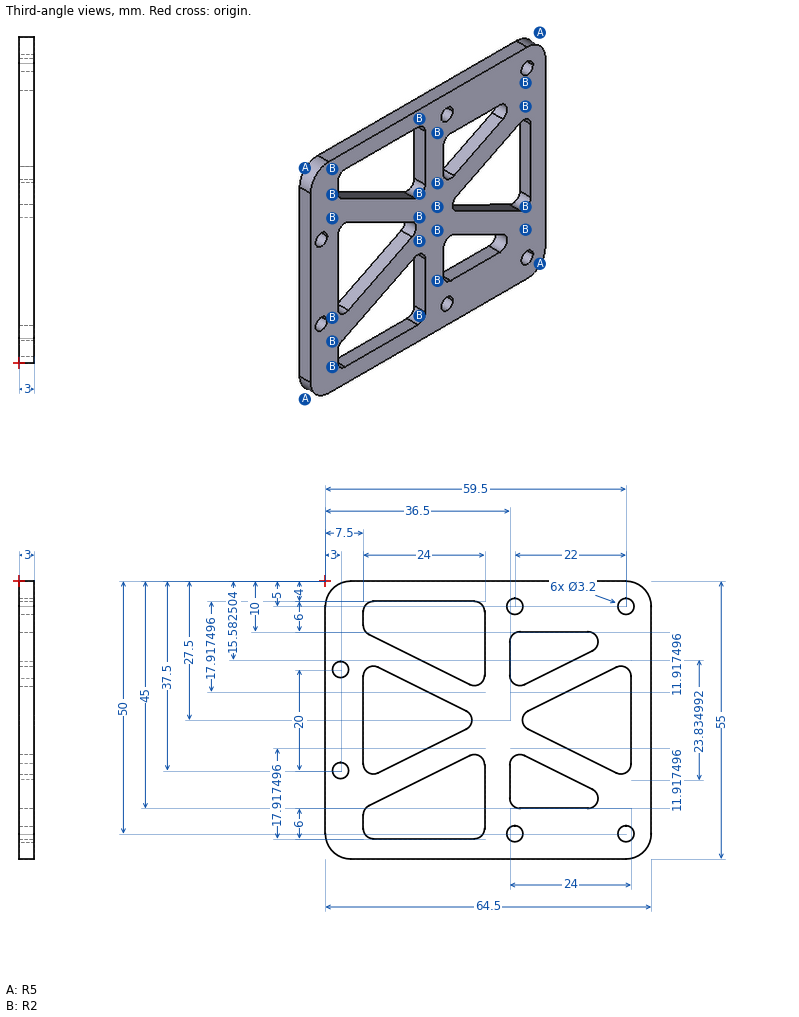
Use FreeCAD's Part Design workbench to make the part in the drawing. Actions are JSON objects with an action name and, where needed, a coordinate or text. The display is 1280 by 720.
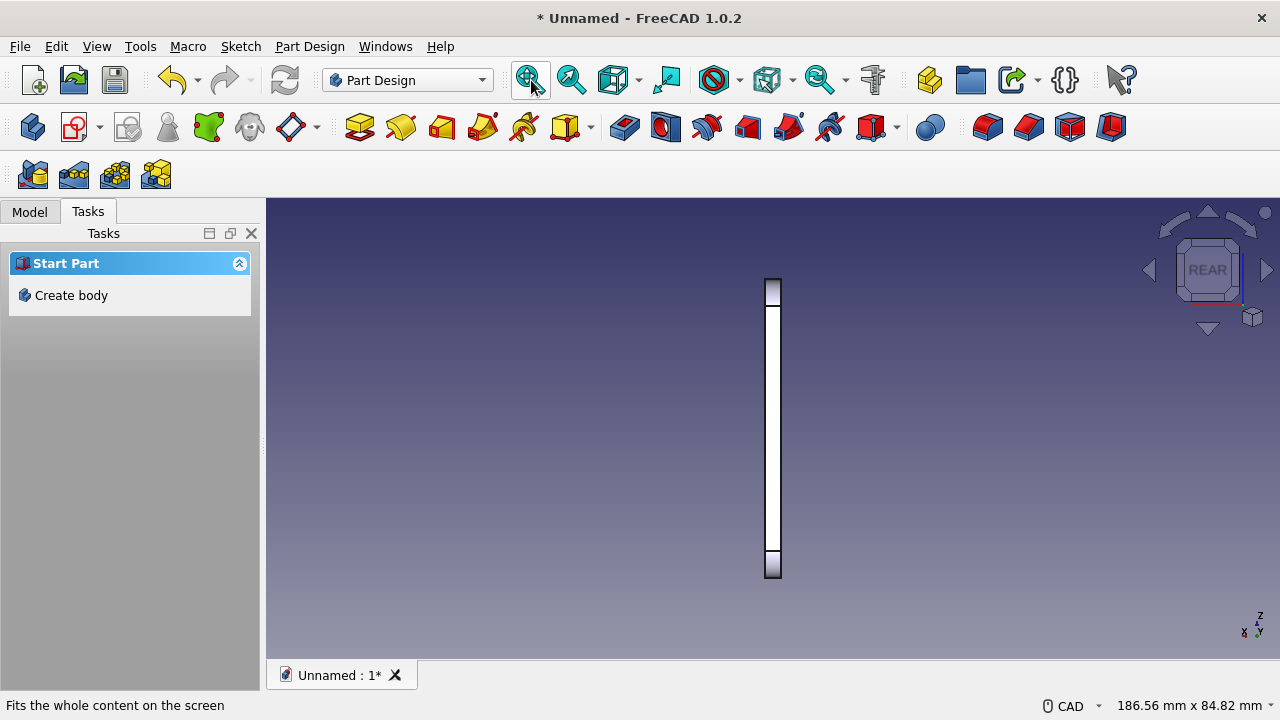
{"action": "scroll", "coordinate": [619, 523], "scroll_direction": "up", "scroll_amount": 5}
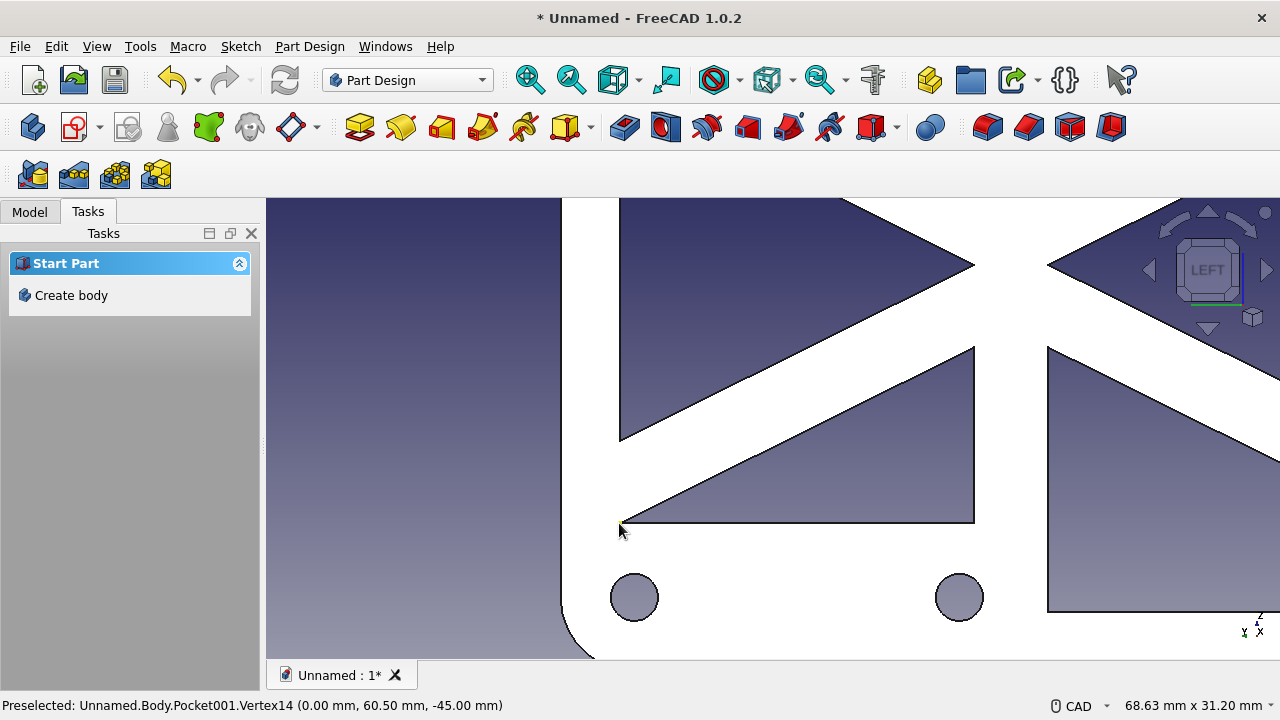
{"action": "key", "text": "v f"}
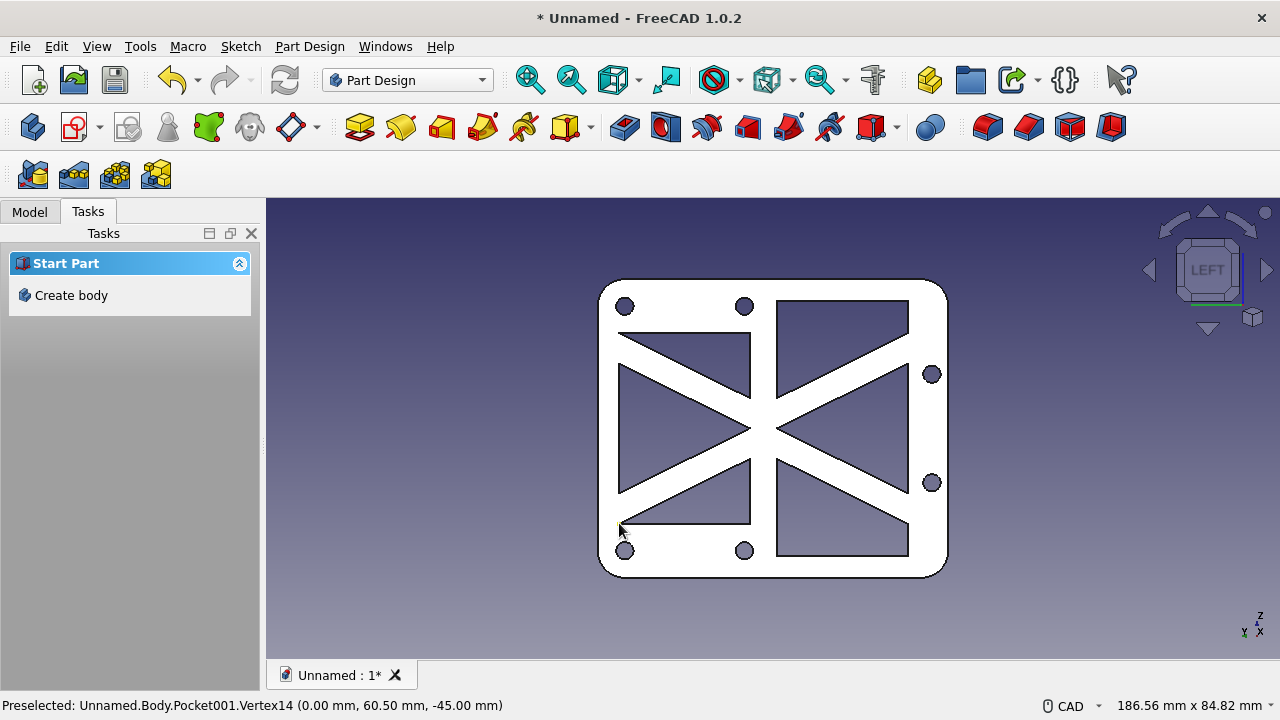
{"action": "key", "text": "v 3"}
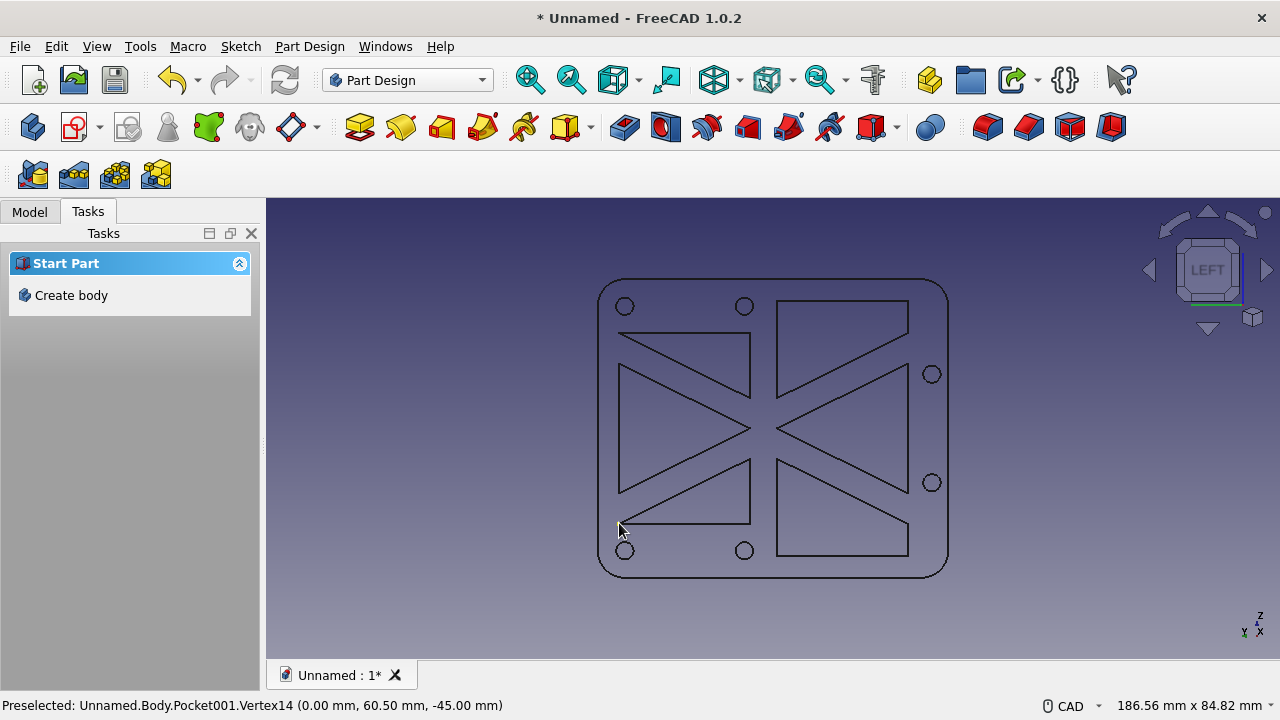
{"action": "key", "text": "0"}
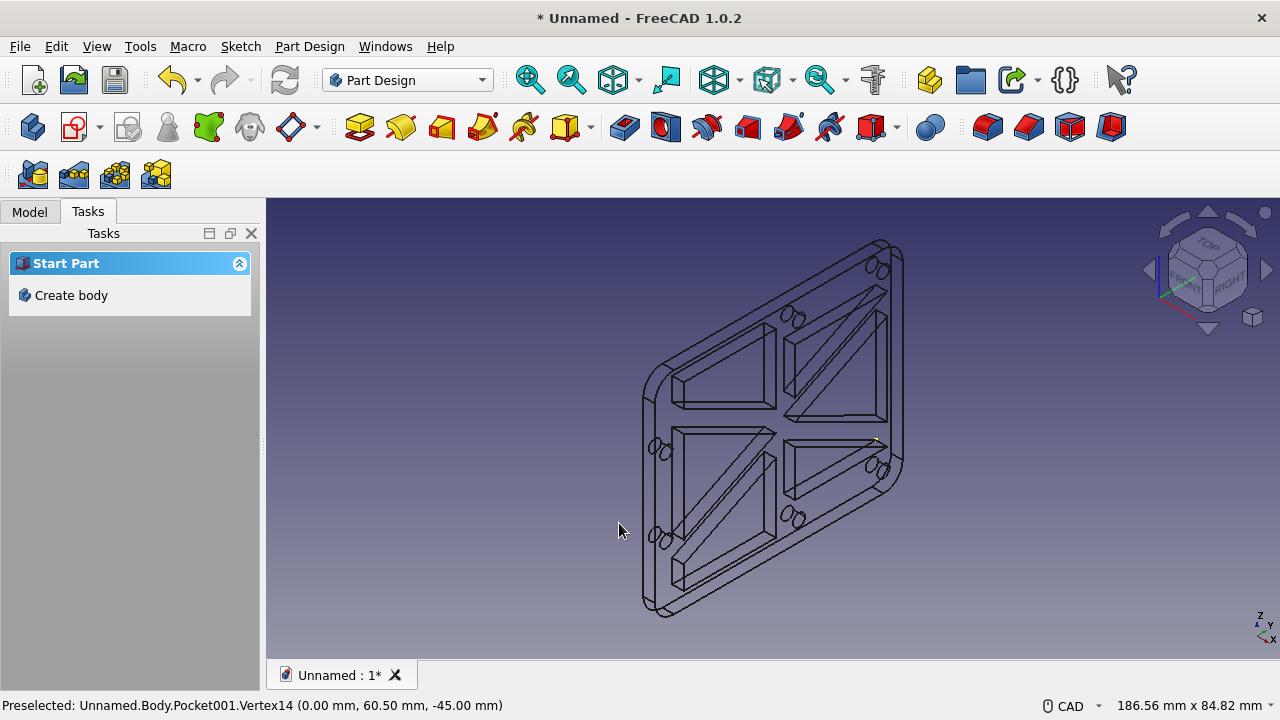
{"action": "left_click", "coordinate": [789, 443]}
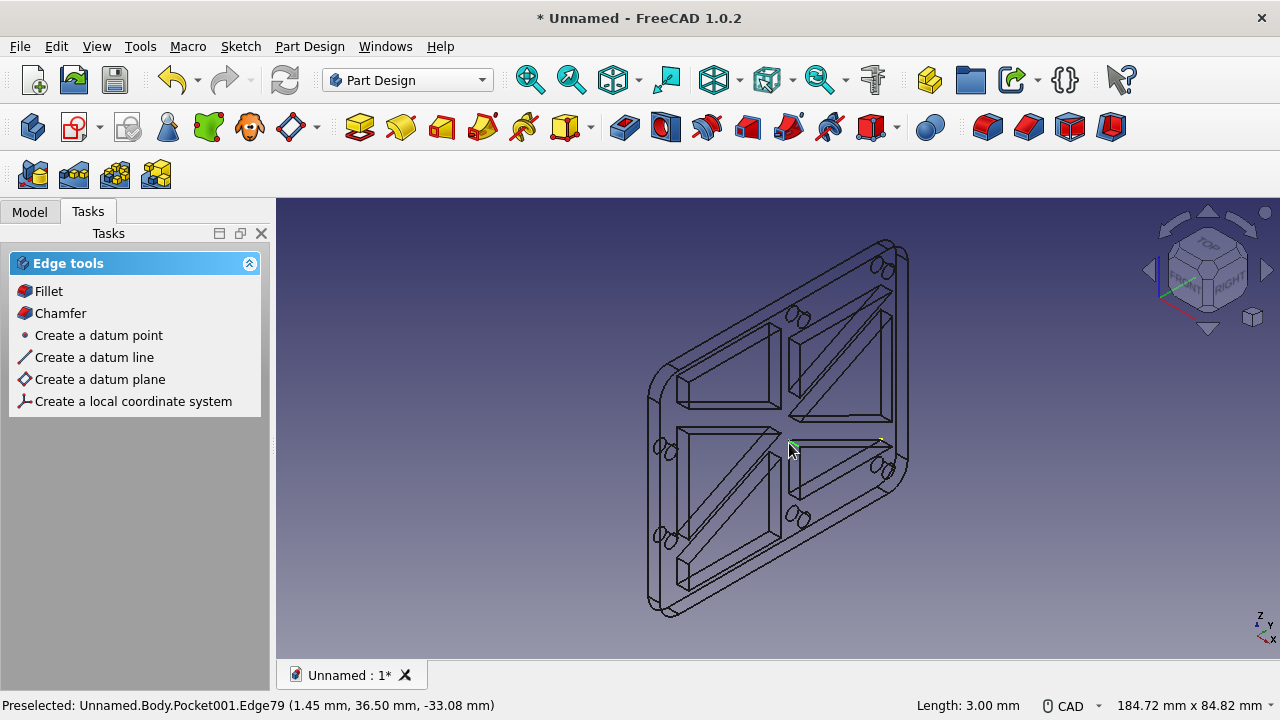
{"action": "left_click", "coordinate": [794, 496], "text": "ctrl"}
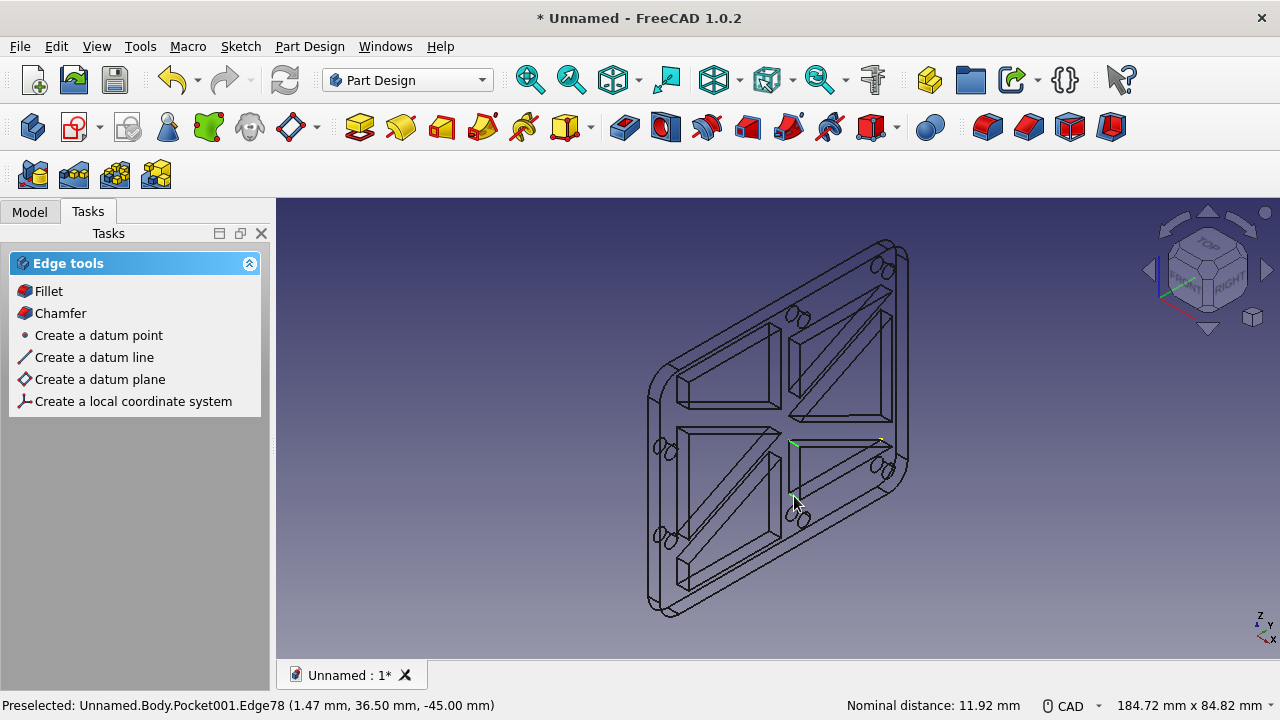
{"action": "left_click", "coordinate": [885, 311], "text": "ctrl"}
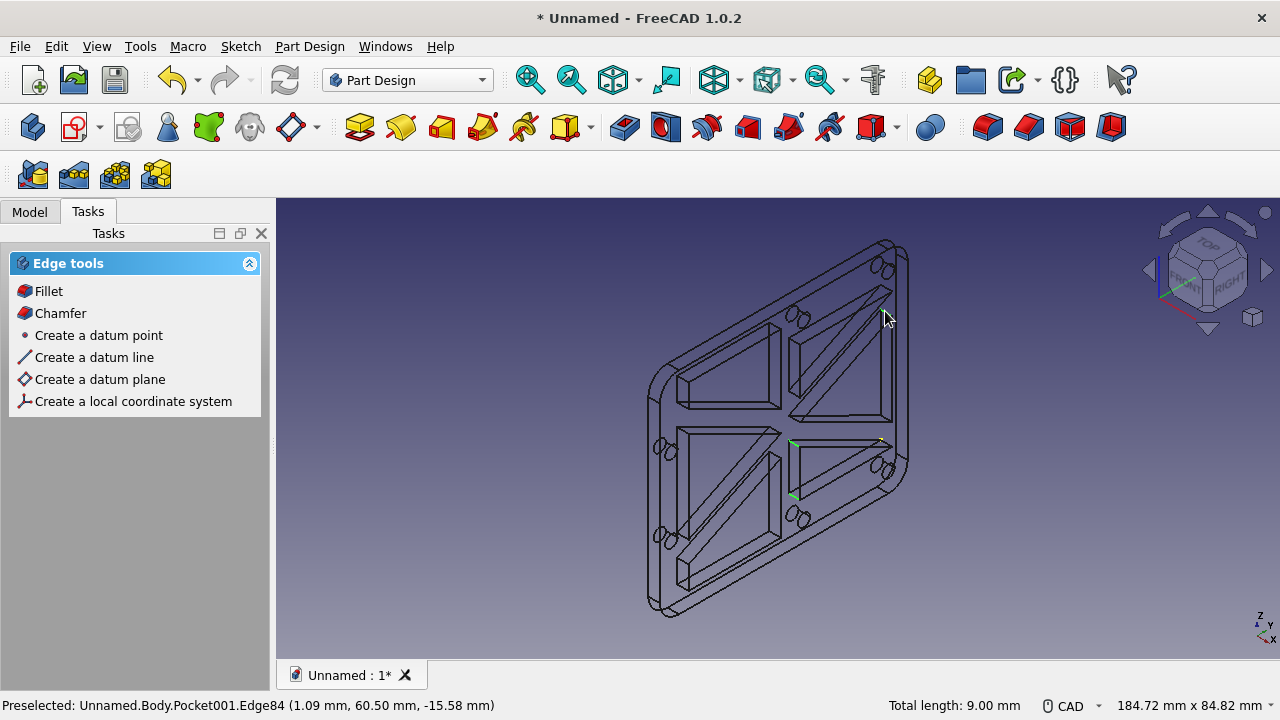
{"action": "left_click", "coordinate": [794, 418], "text": "ctrl"}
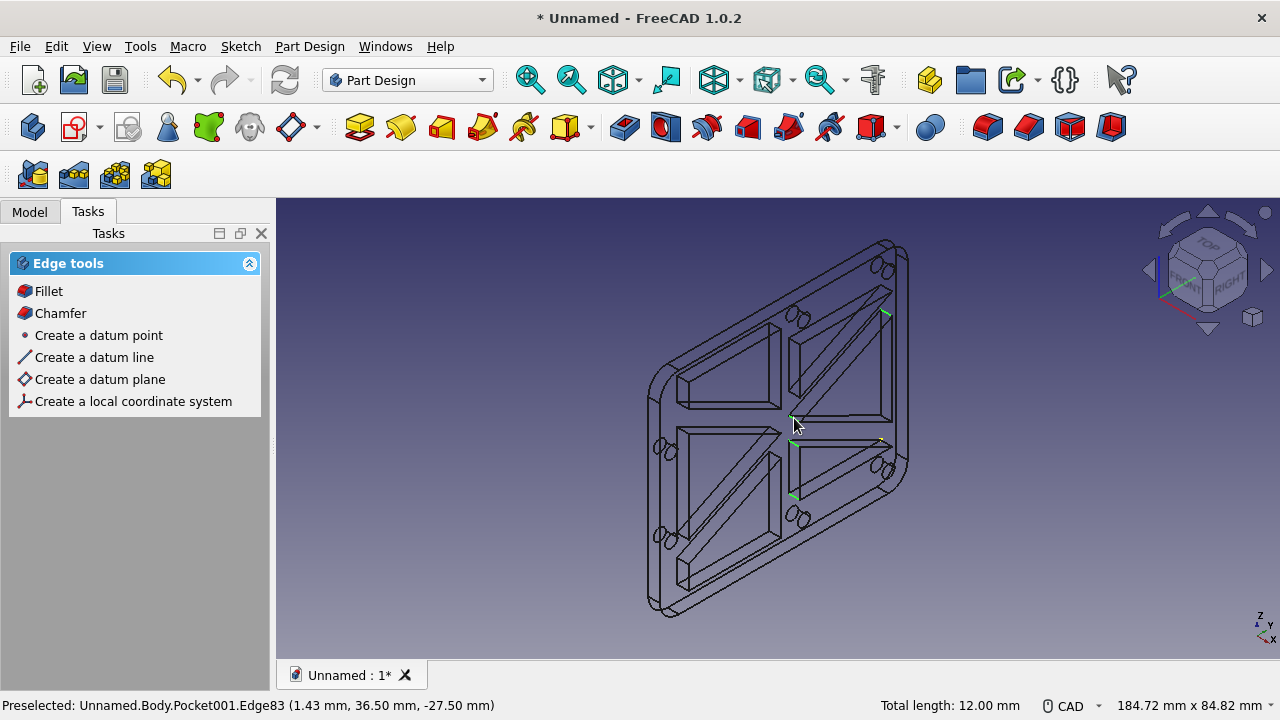
{"action": "left_click", "coordinate": [683, 430], "text": "ctrl"}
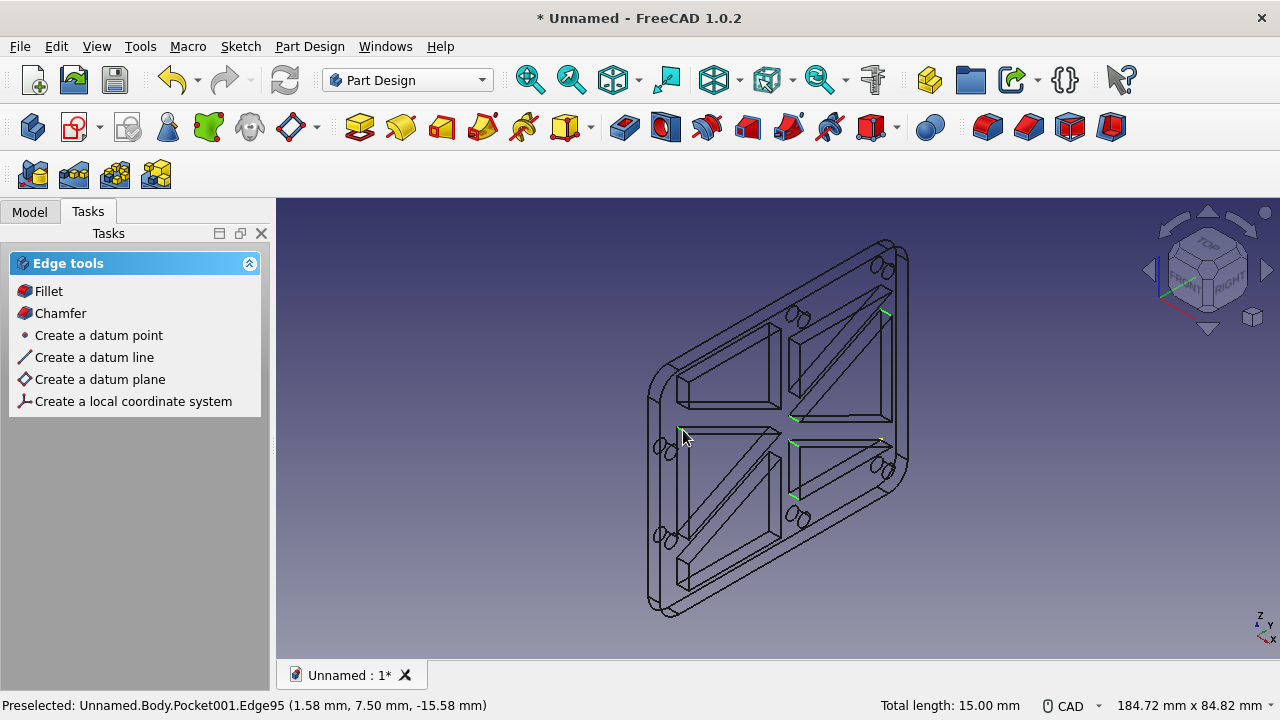
{"action": "left_click", "coordinate": [774, 324], "text": "ctrl"}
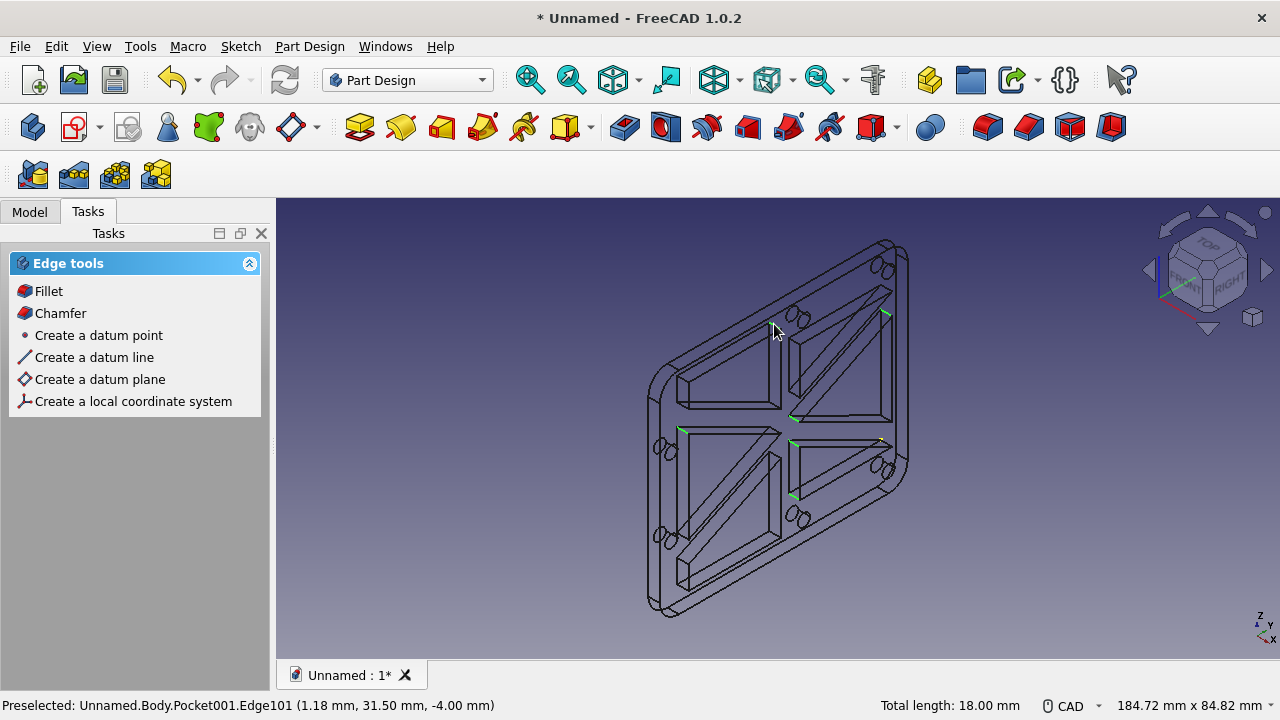
{"action": "left_click", "coordinate": [683, 378], "text": "ctrl"}